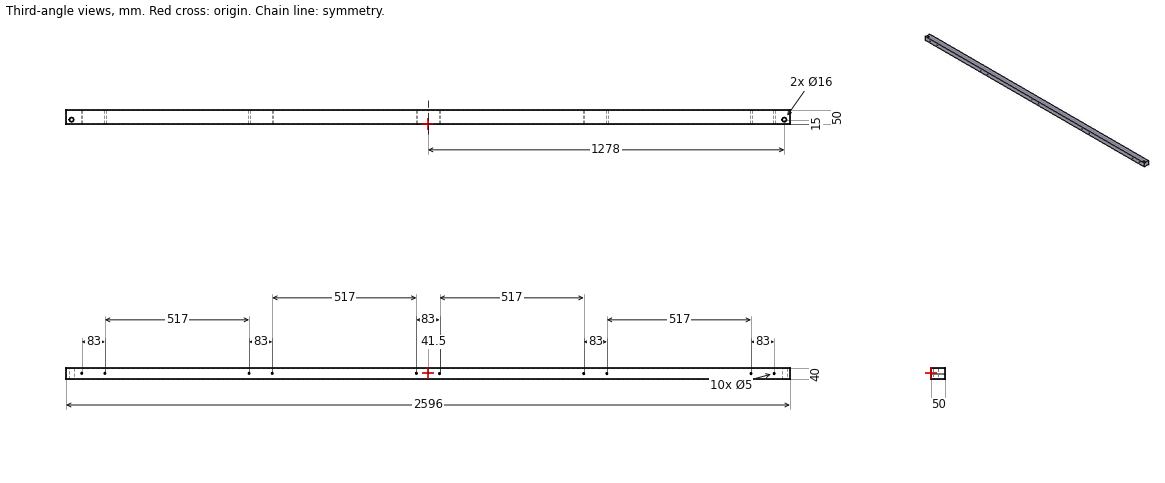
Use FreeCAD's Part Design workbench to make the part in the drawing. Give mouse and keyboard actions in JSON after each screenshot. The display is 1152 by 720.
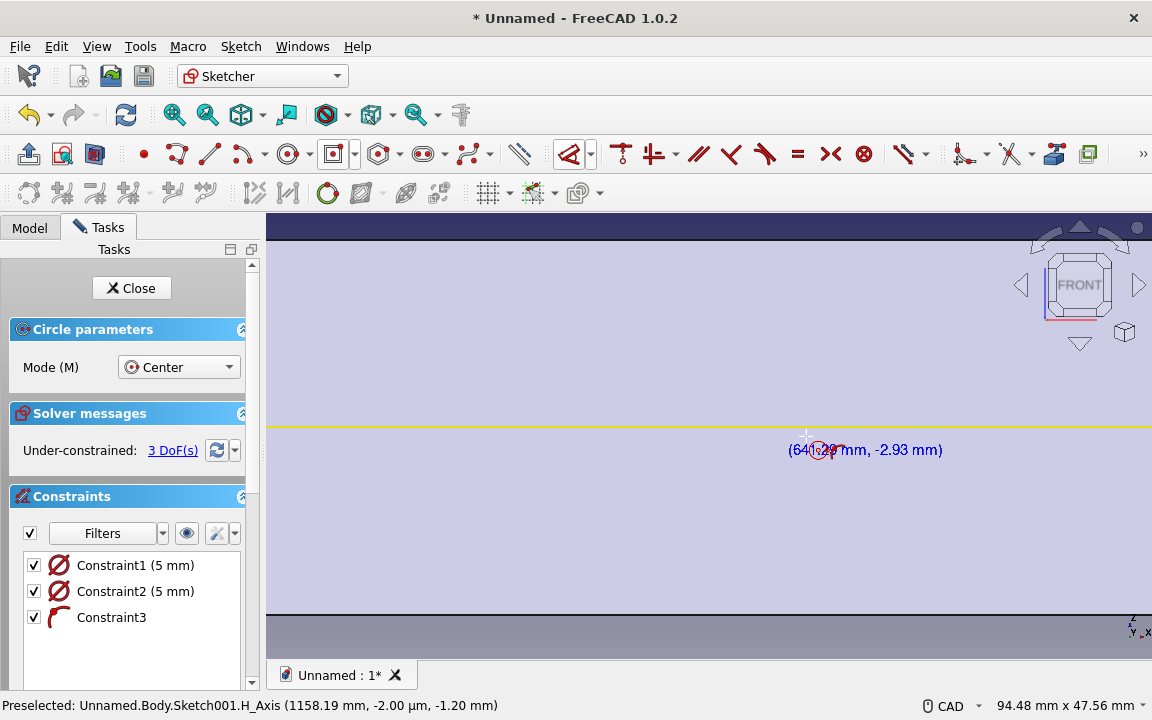
{"action": "scroll", "coordinate": [805, 436], "scroll_direction": "down", "scroll_amount": 18}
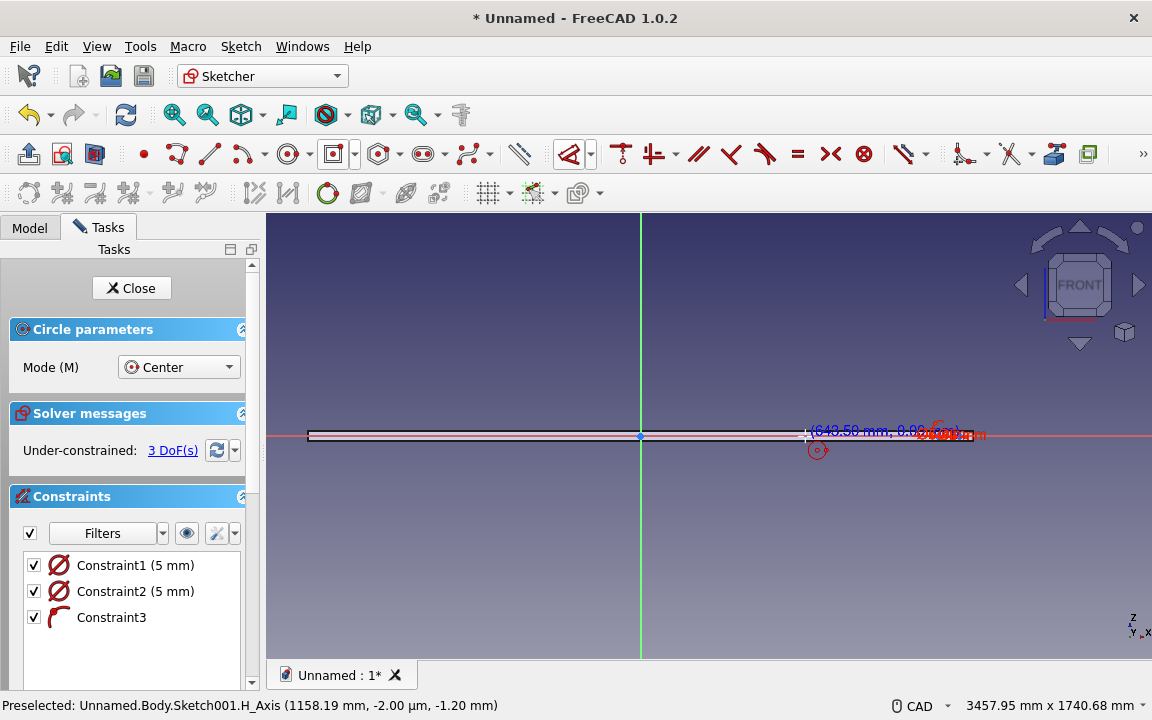
{"action": "left_click", "coordinate": [805, 436]}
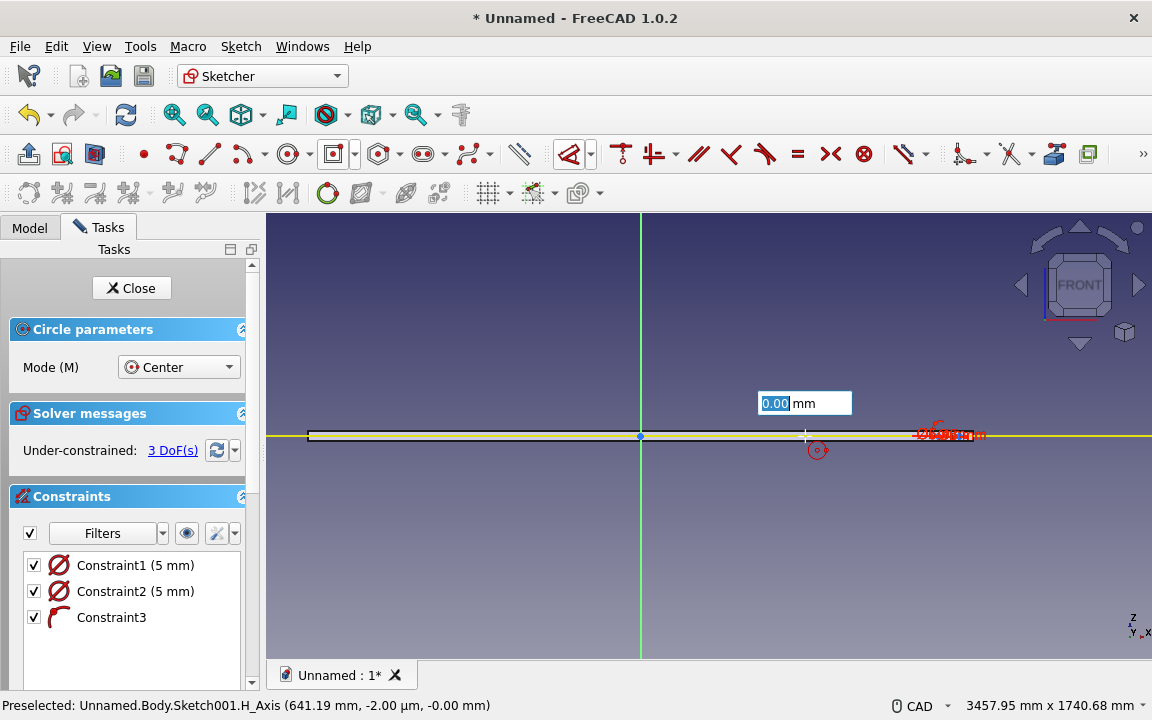
{"action": "scroll", "coordinate": [805, 437], "scroll_direction": "up", "scroll_amount": 17}
{"action": "mouse_move", "coordinate": [783, 418]}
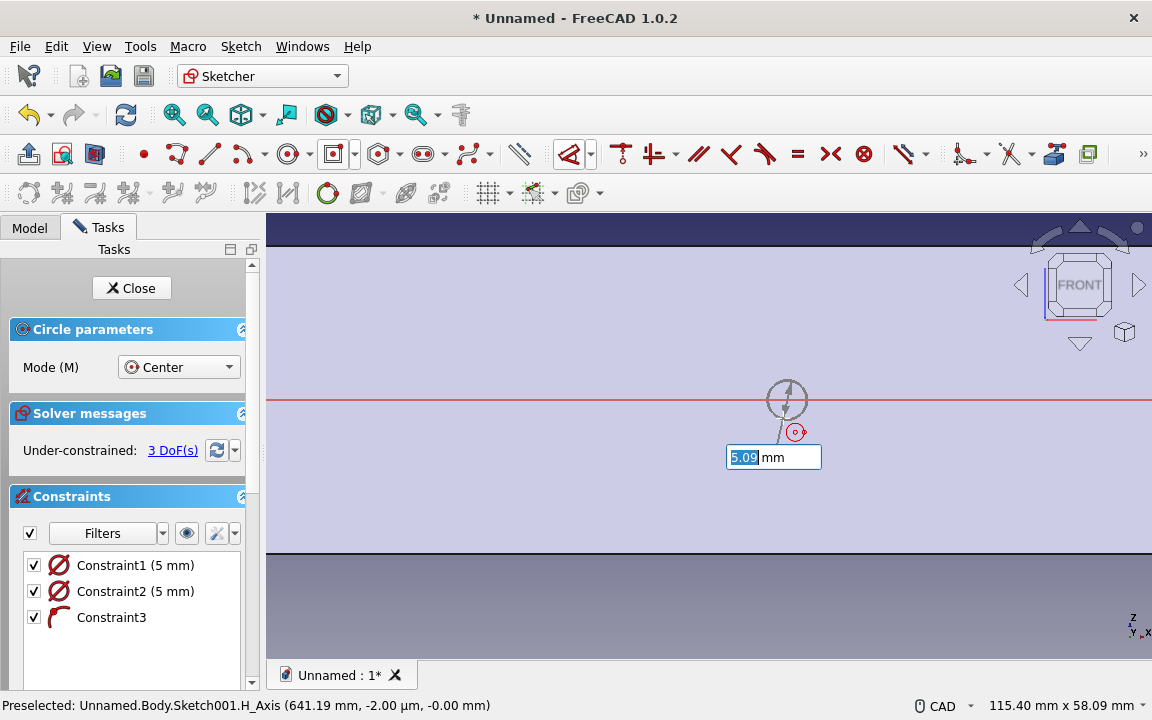
{"action": "type", "text": "5"}
{"action": "key", "text": "Return"}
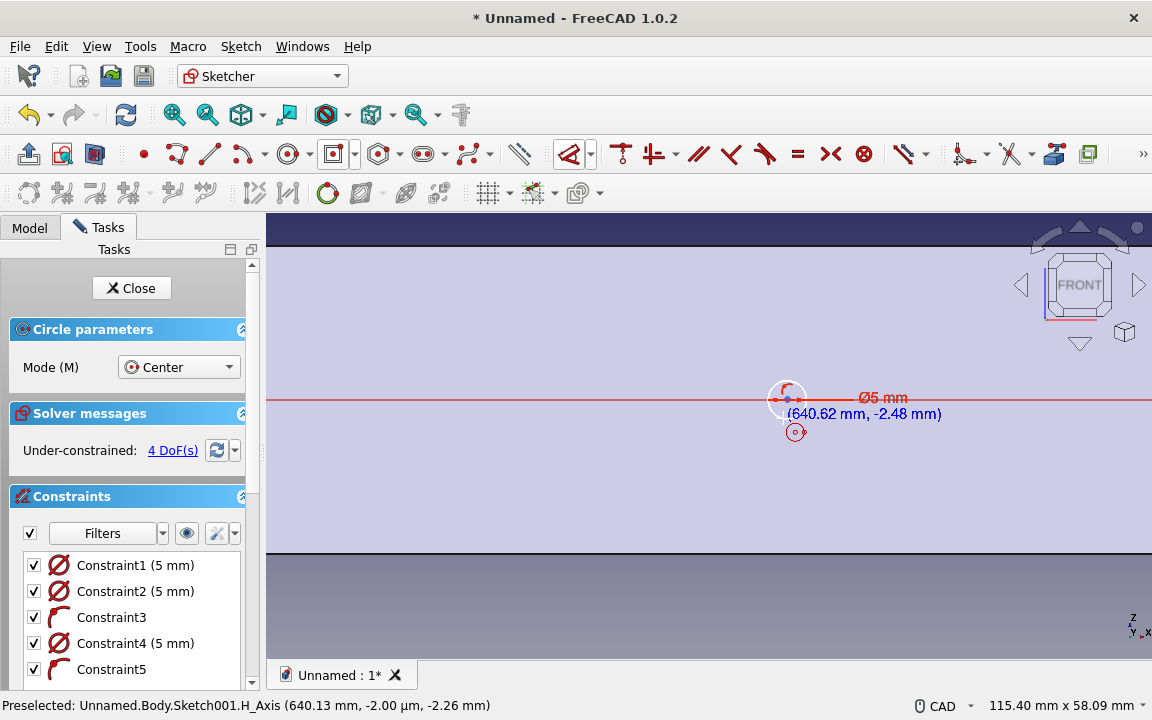
{"action": "scroll", "coordinate": [805, 437], "scroll_direction": "down", "scroll_amount": 17}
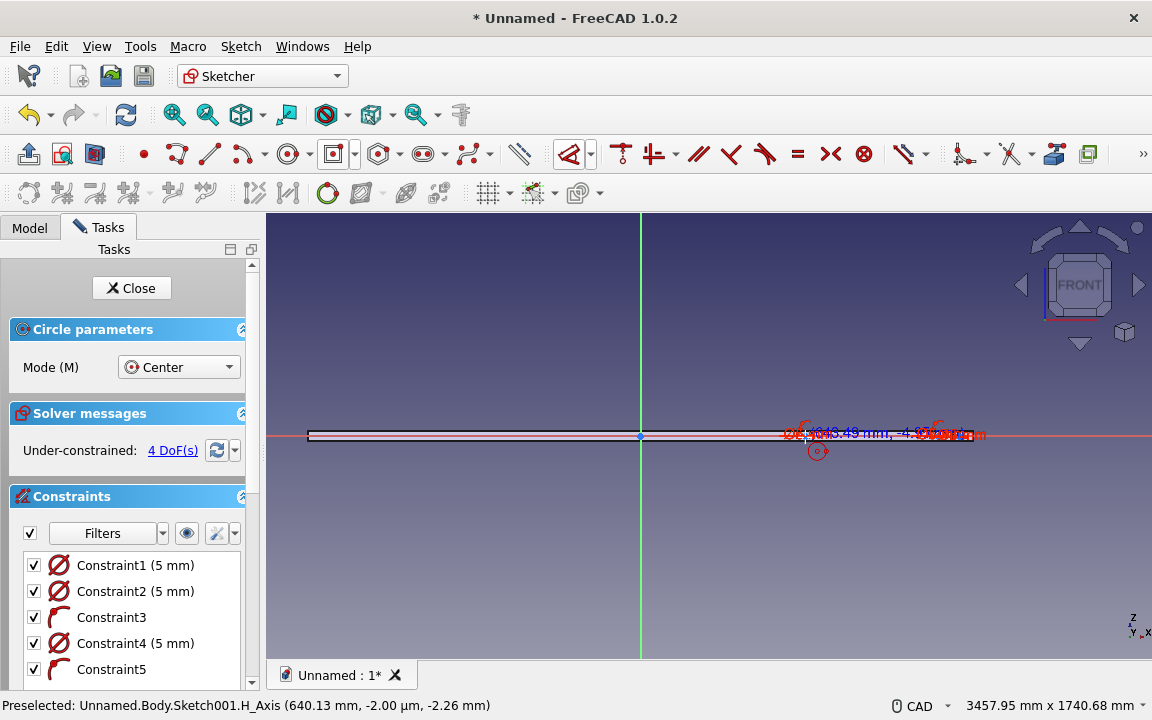
{"action": "scroll", "coordinate": [784, 436], "scroll_direction": "up", "scroll_amount": 18}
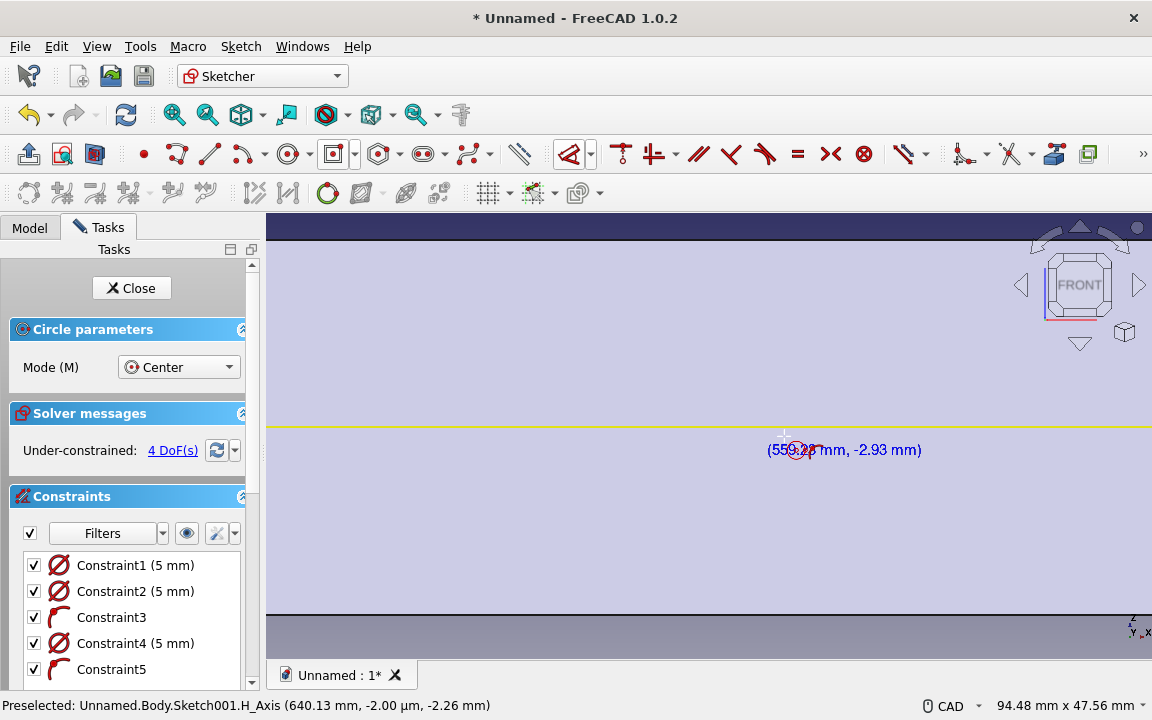
{"action": "scroll", "coordinate": [784, 436], "scroll_direction": "down", "scroll_amount": 18}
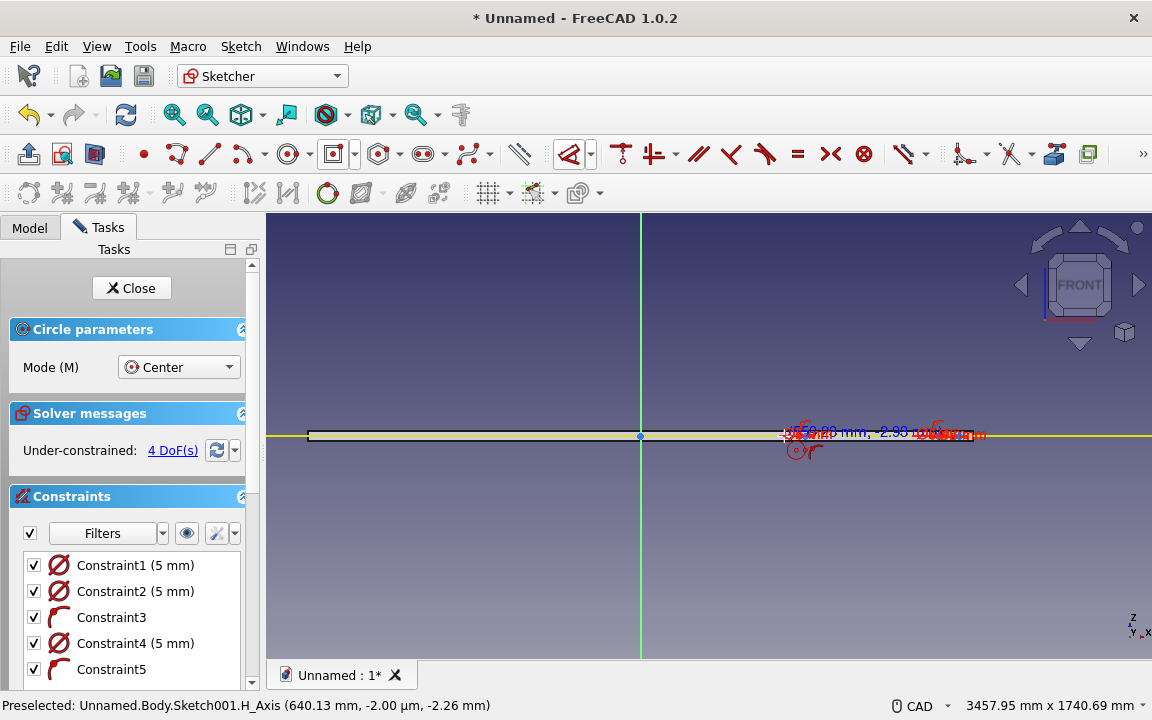
{"action": "left_click", "coordinate": [784, 436]}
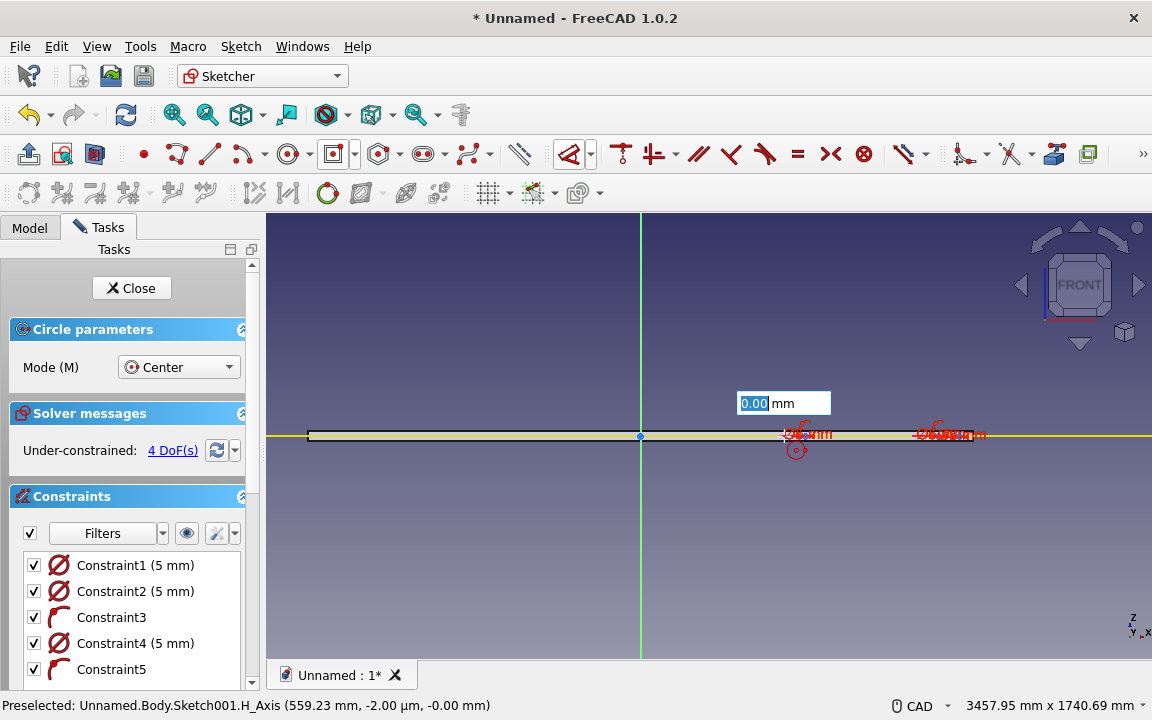
{"action": "scroll", "coordinate": [784, 437], "scroll_direction": "up", "scroll_amount": 17}
{"action": "mouse_move", "coordinate": [755, 418]}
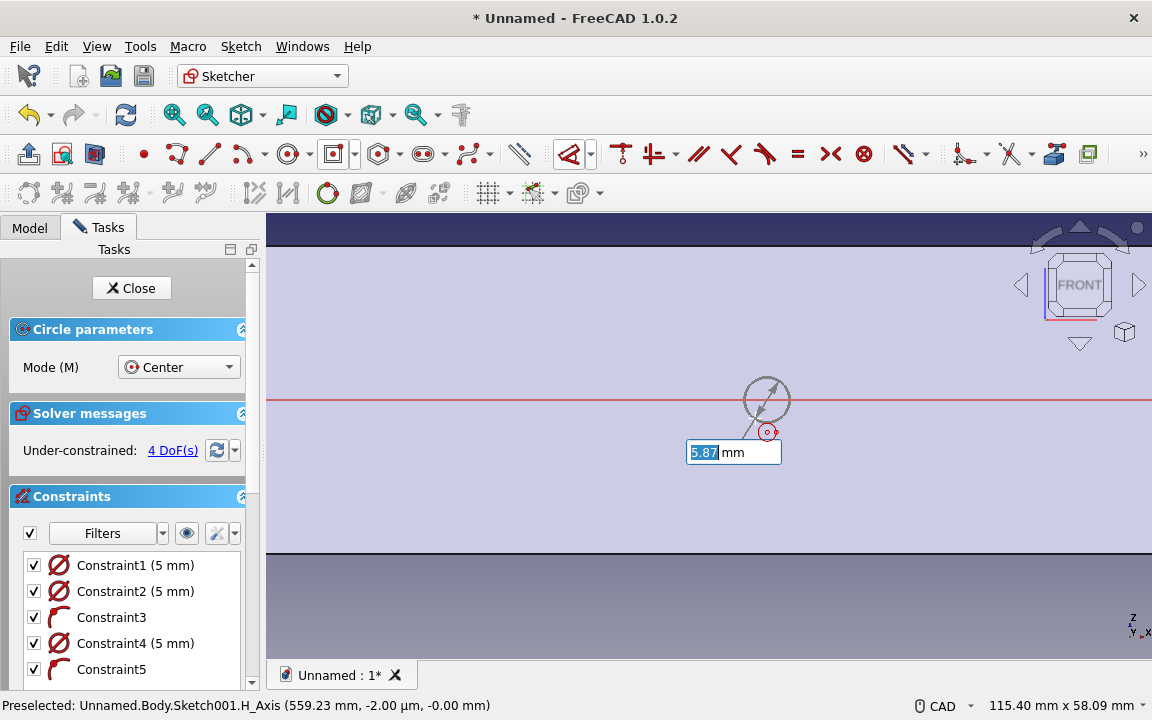
{"action": "type", "text": "5"}
{"action": "key", "text": "Return"}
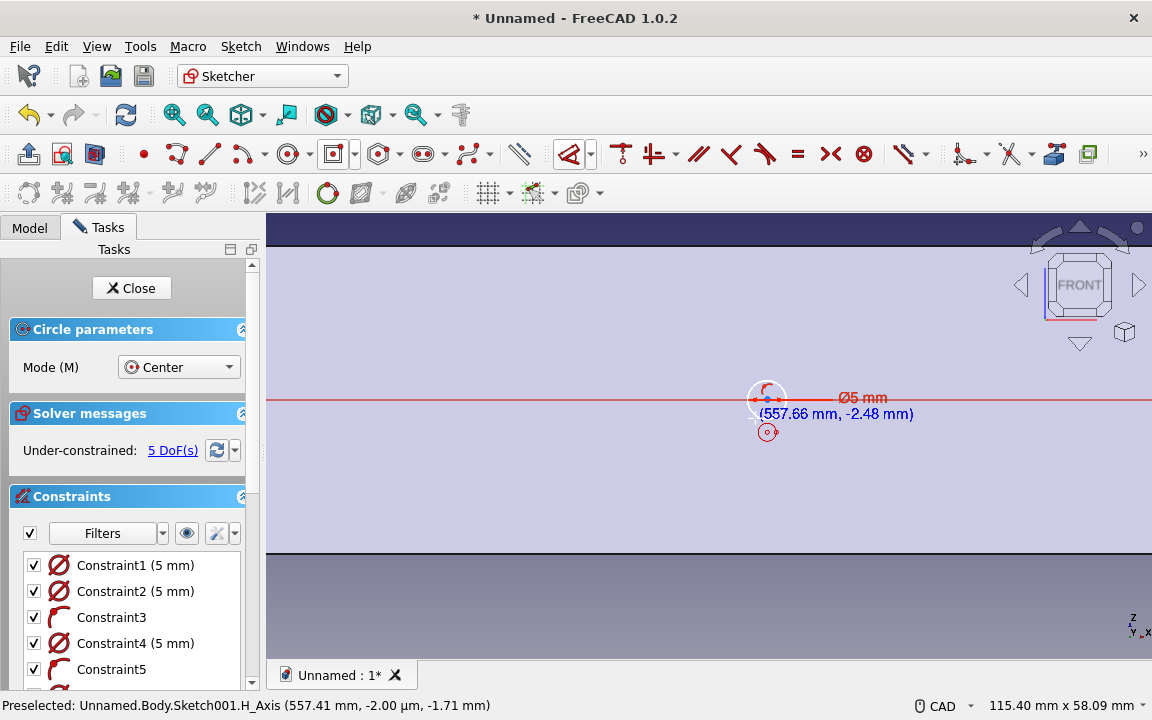
{"action": "scroll", "coordinate": [784, 437], "scroll_direction": "down", "scroll_amount": 17}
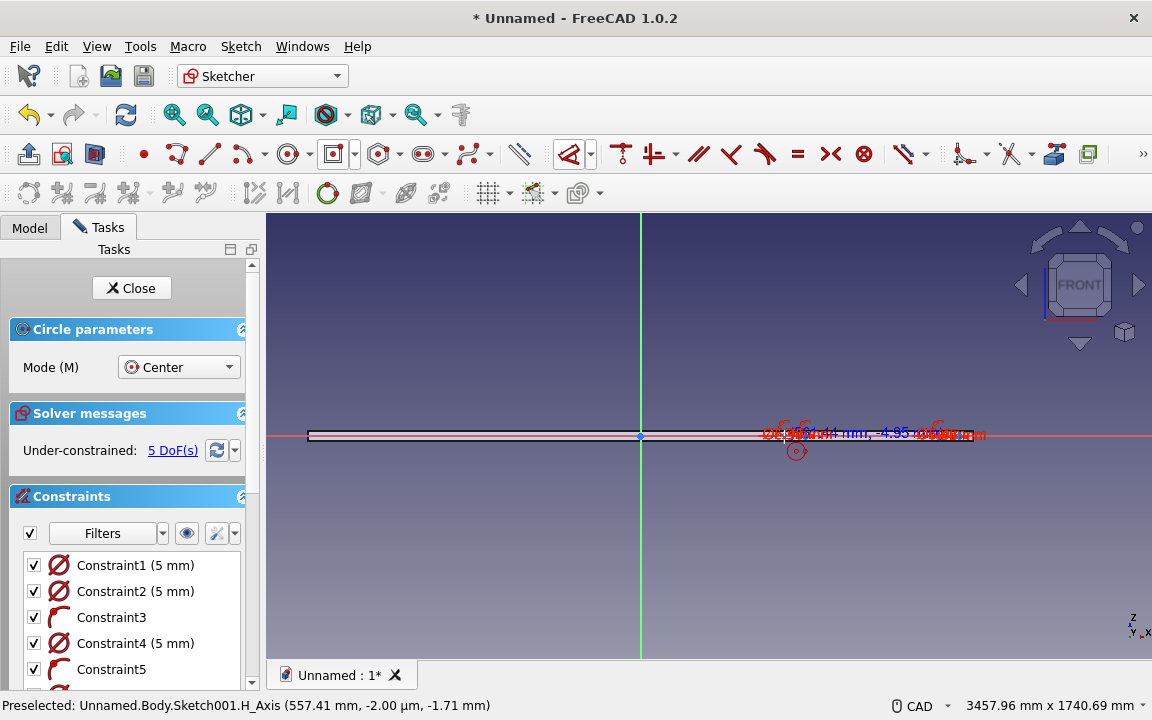
{"action": "scroll", "coordinate": [651, 436], "scroll_direction": "up", "scroll_amount": 18}